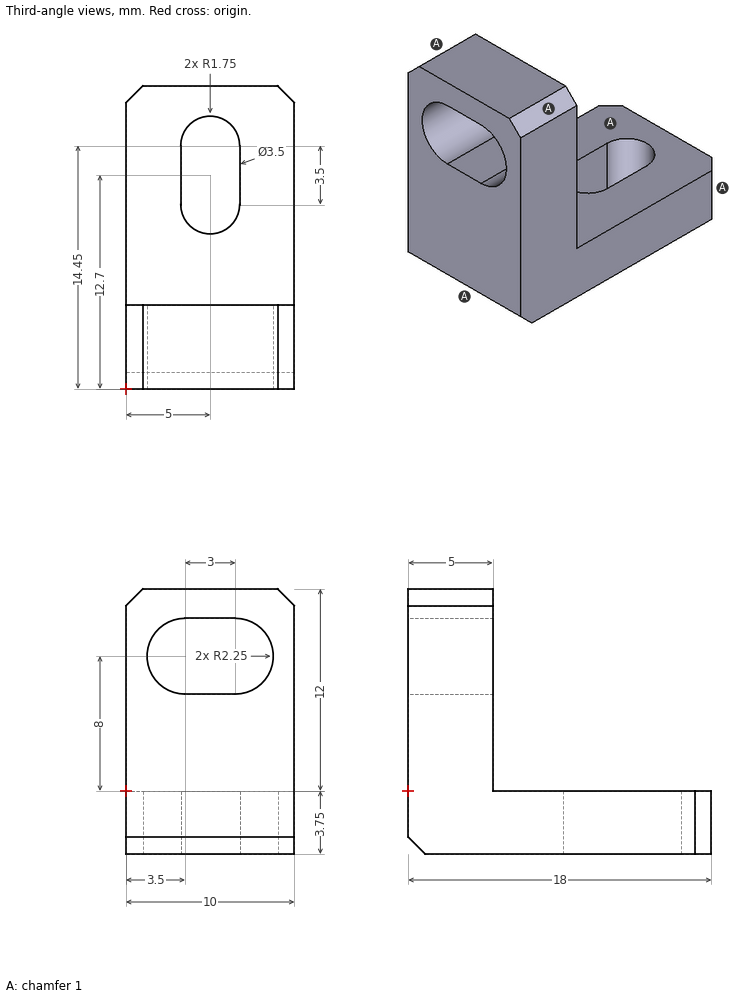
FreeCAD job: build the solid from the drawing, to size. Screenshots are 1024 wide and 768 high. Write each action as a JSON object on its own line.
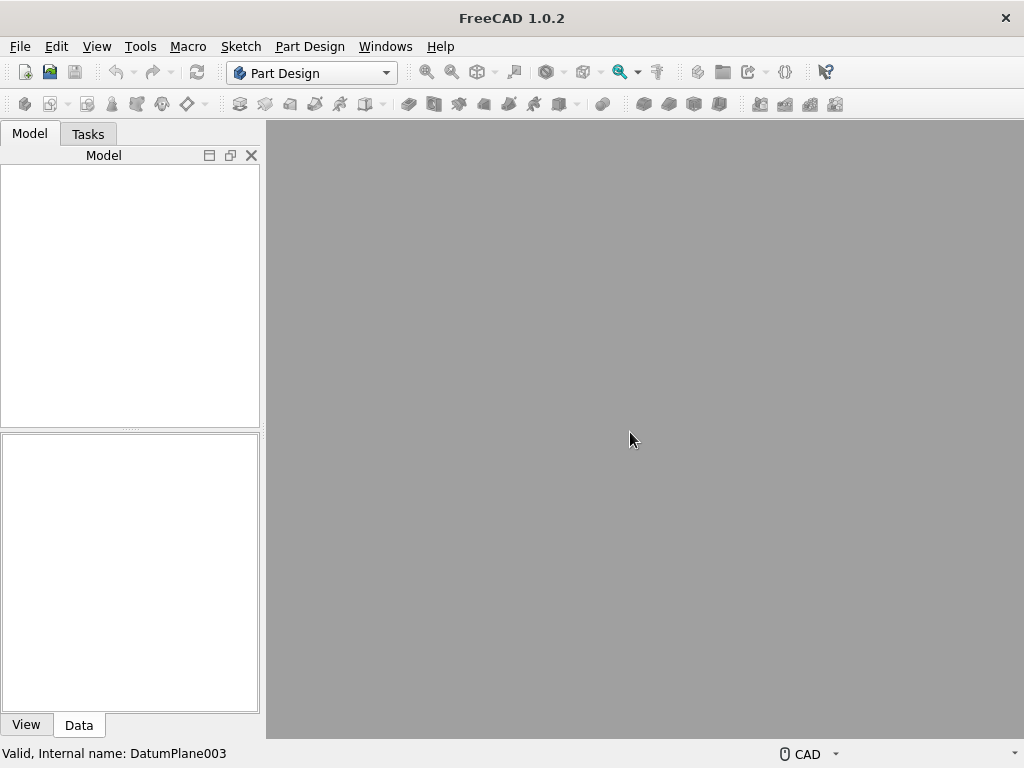
{"action": "left_click", "coordinate": [25, 72]}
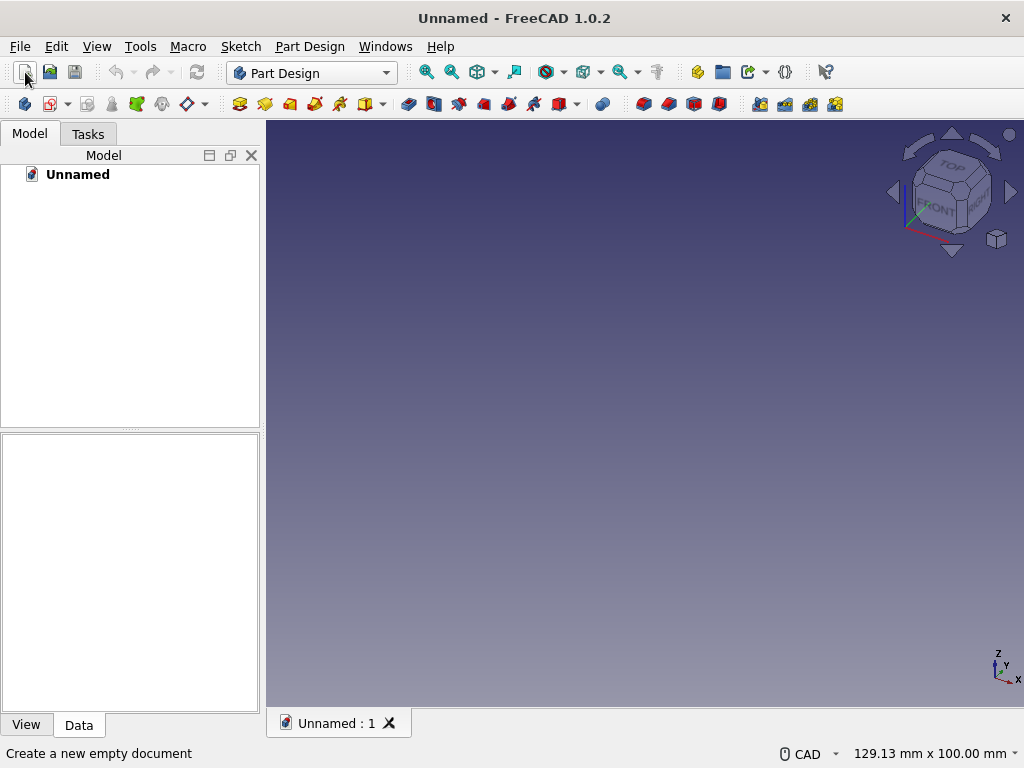
{"action": "left_click", "coordinate": [50, 104]}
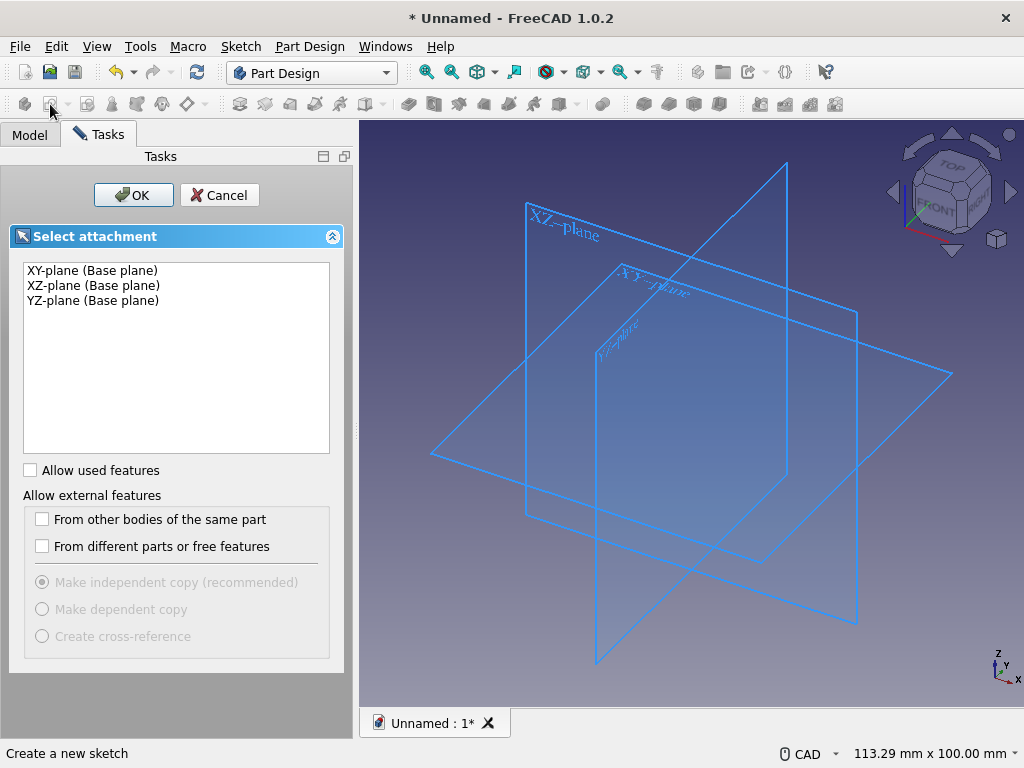
{"action": "left_click", "coordinate": [84, 286]}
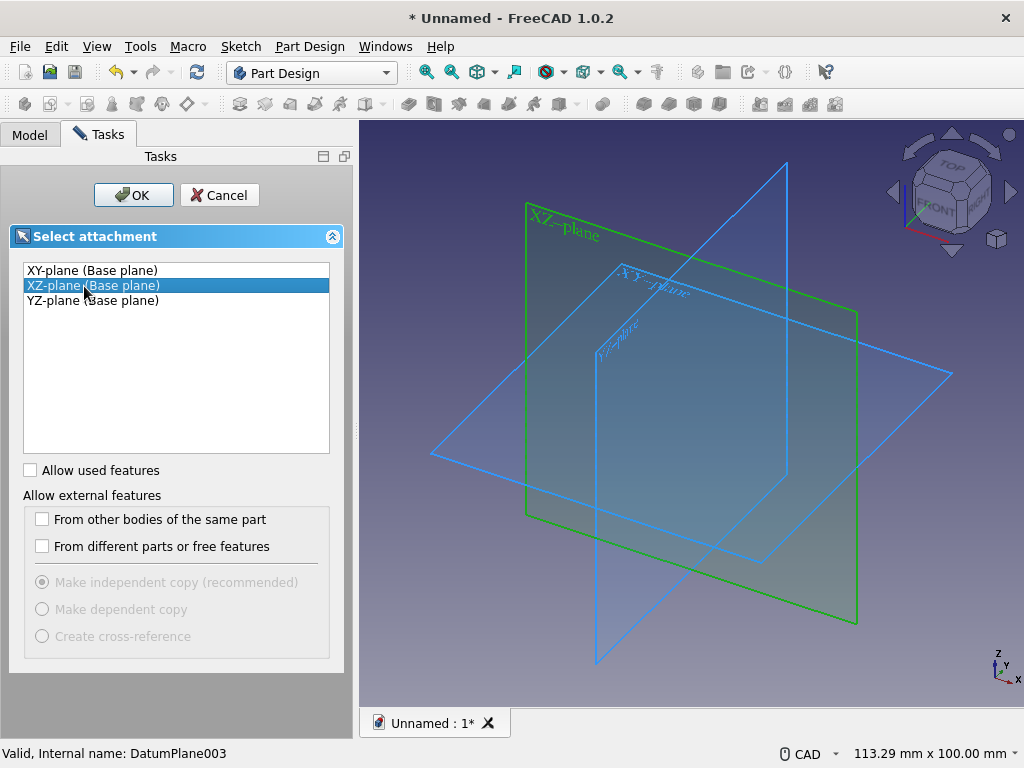
{"action": "left_click", "coordinate": [134, 195]}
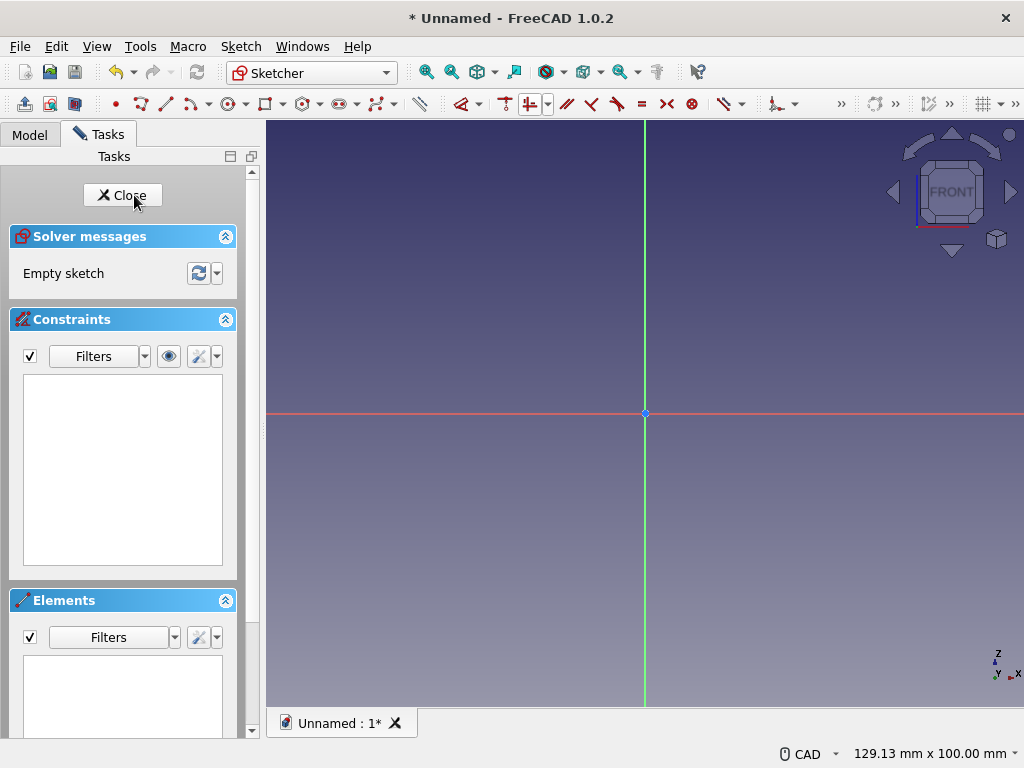
{"action": "scroll", "coordinate": [690, 426], "scroll_direction": "up", "scroll_amount": 10}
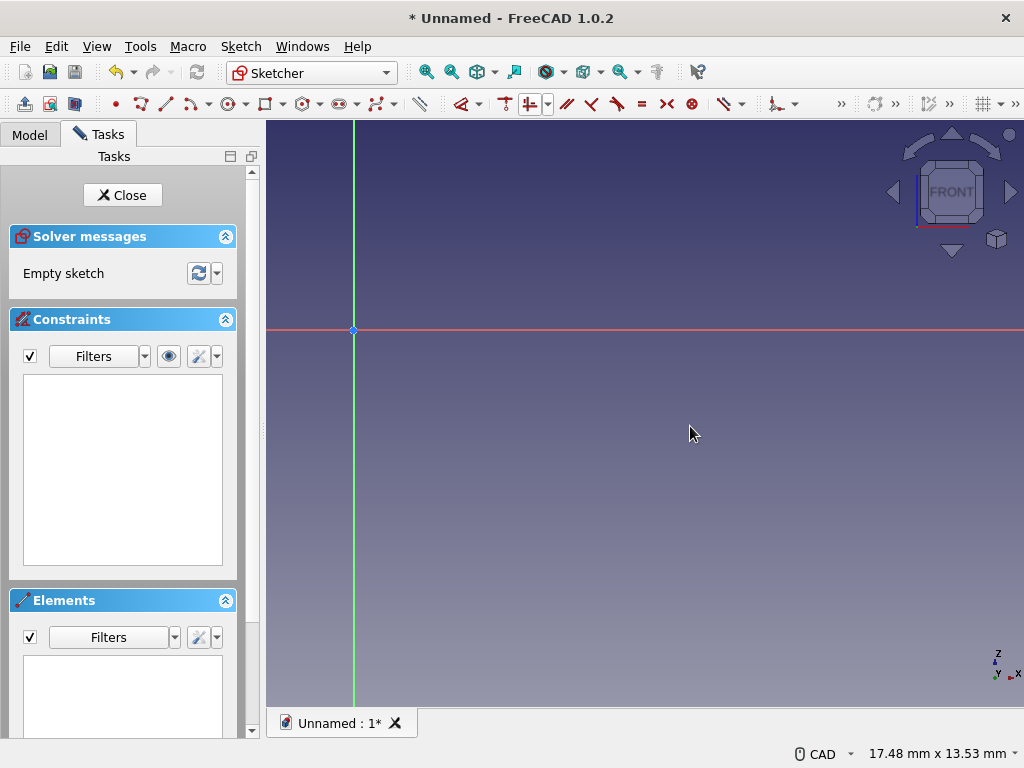
{"action": "key", "text": "g r"}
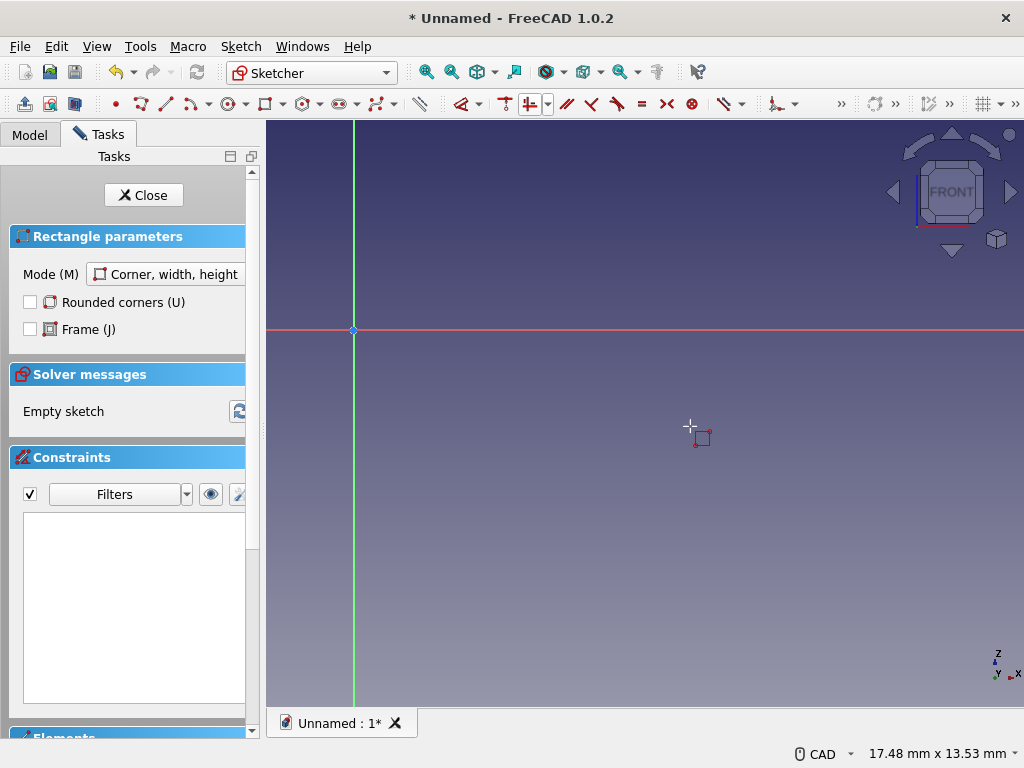
{"action": "left_click", "coordinate": [354, 330]}
{"action": "mouse_move", "coordinate": [788, 493]}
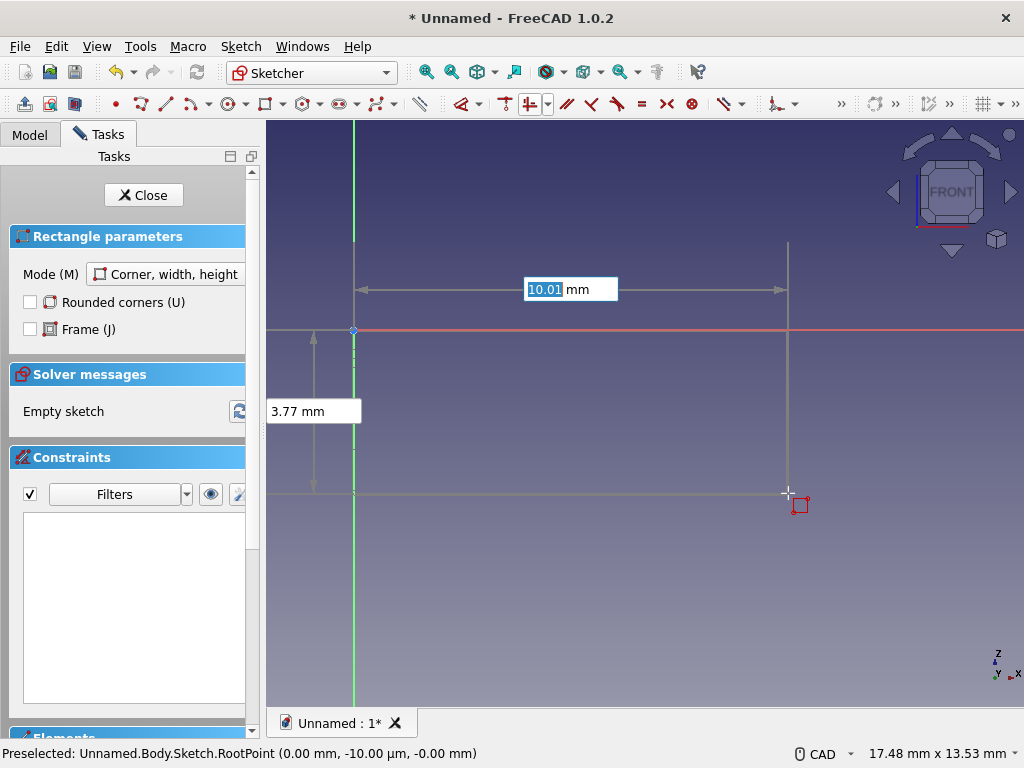
{"action": "type", "text": "10"}
{"action": "key", "text": "Tab"}
{"action": "type", "text": "3.75"}
{"action": "key", "text": "Return"}
{"action": "key", "text": "Escape"}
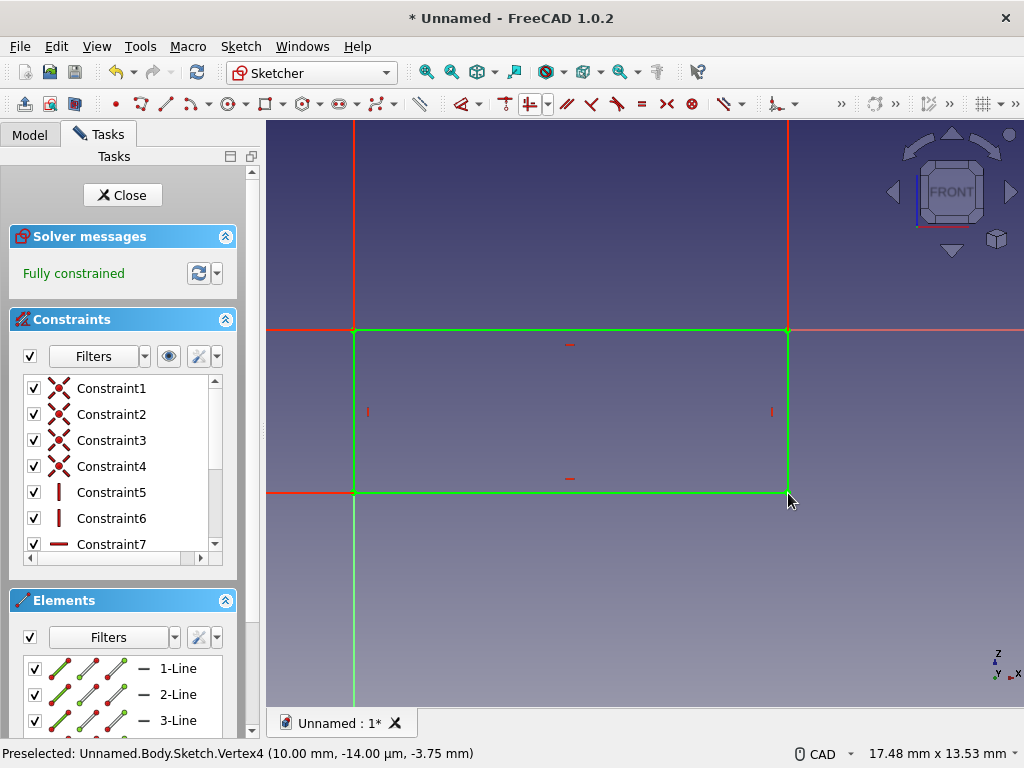
{"action": "left_click", "coordinate": [123, 195]}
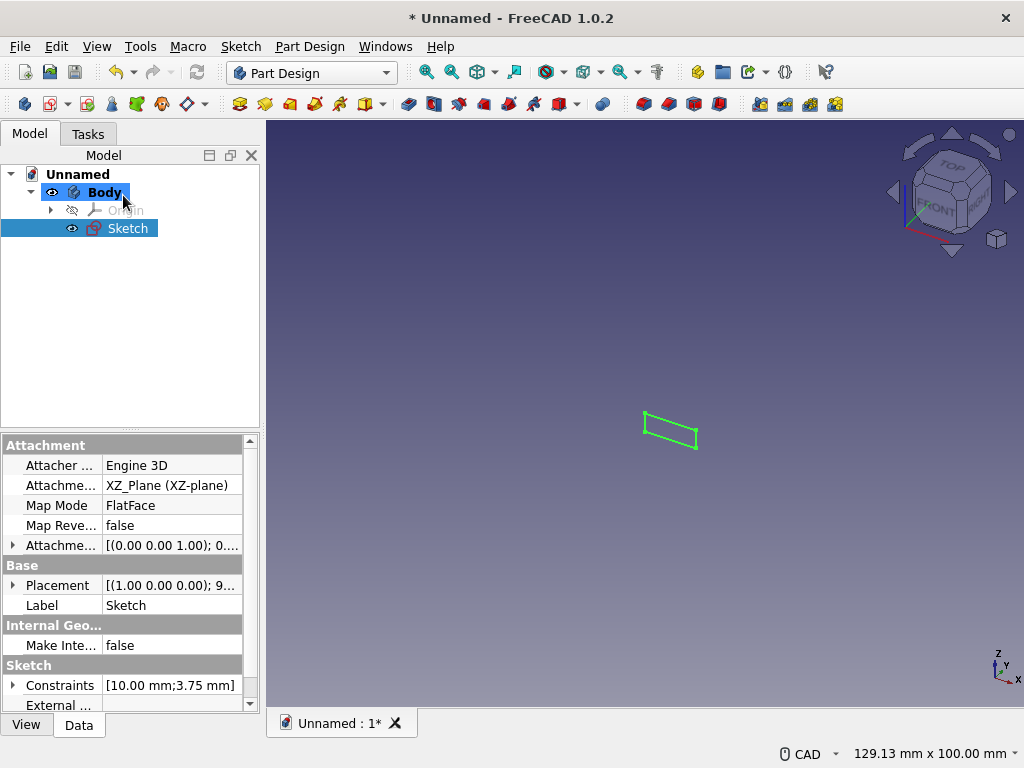
{"action": "left_click", "coordinate": [240, 104]}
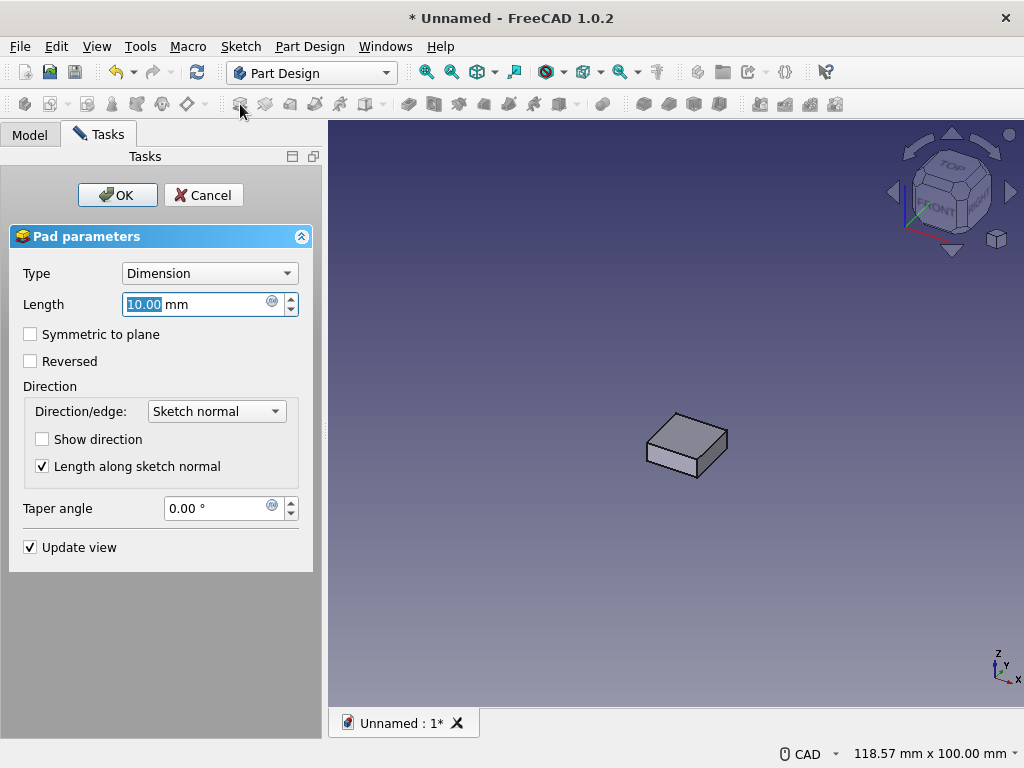
{"action": "type", "text": "18"}
{"action": "key", "text": "Tab"}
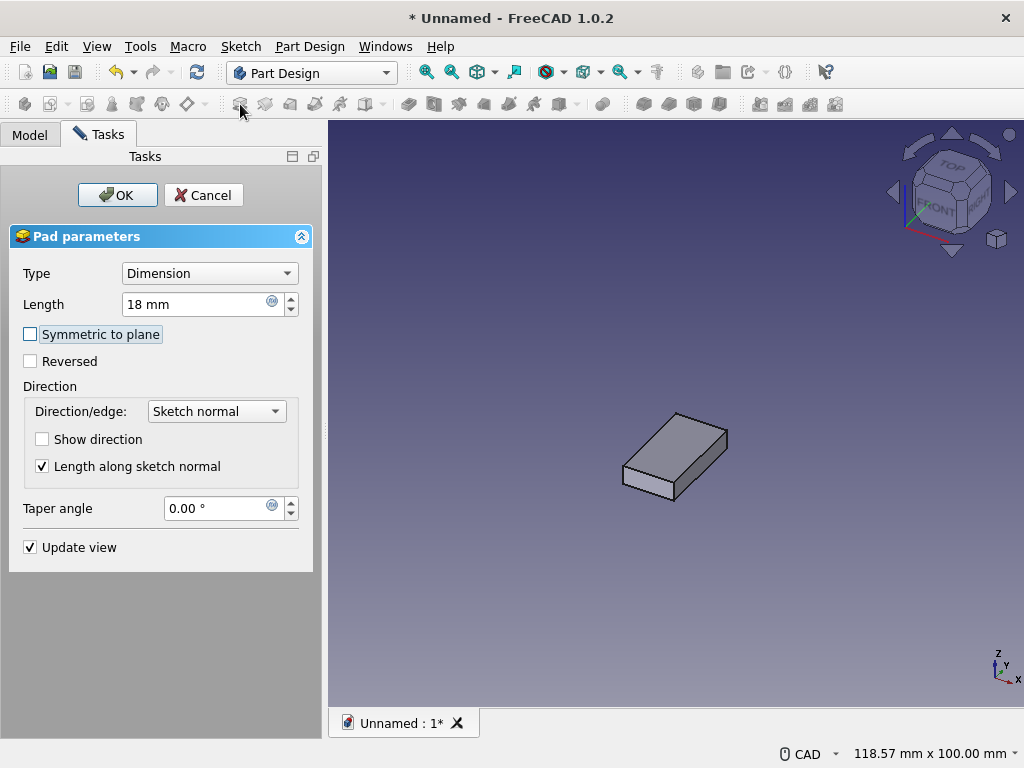
{"action": "left_click", "coordinate": [31, 361]}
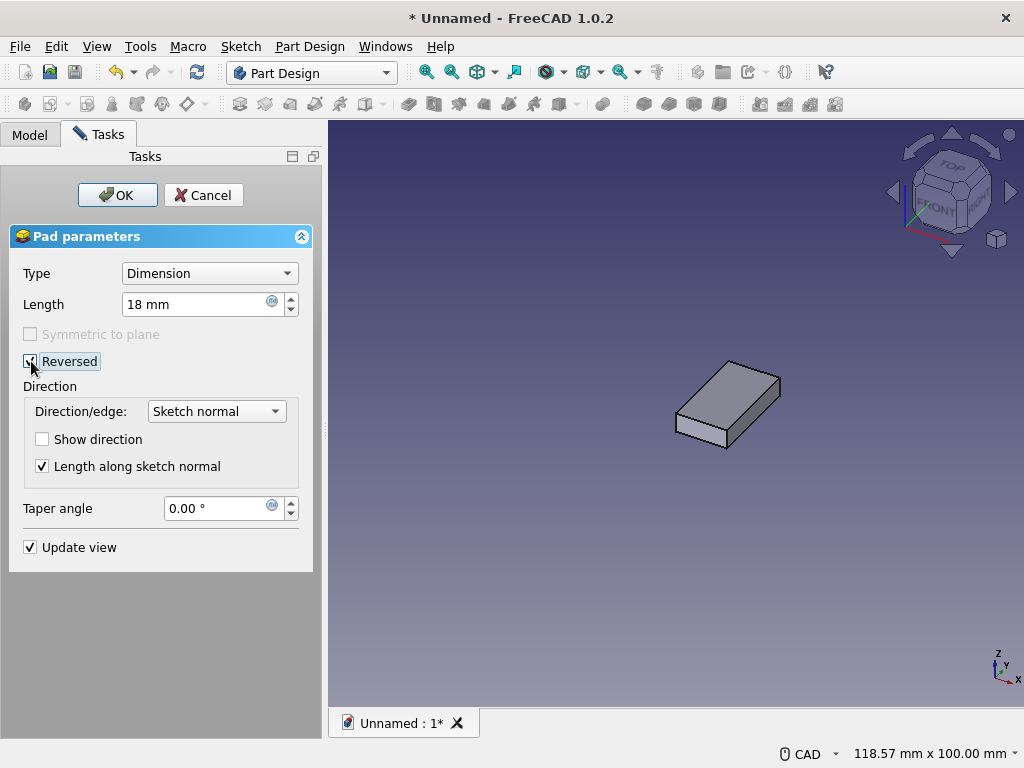
{"action": "left_click", "coordinate": [118, 195]}